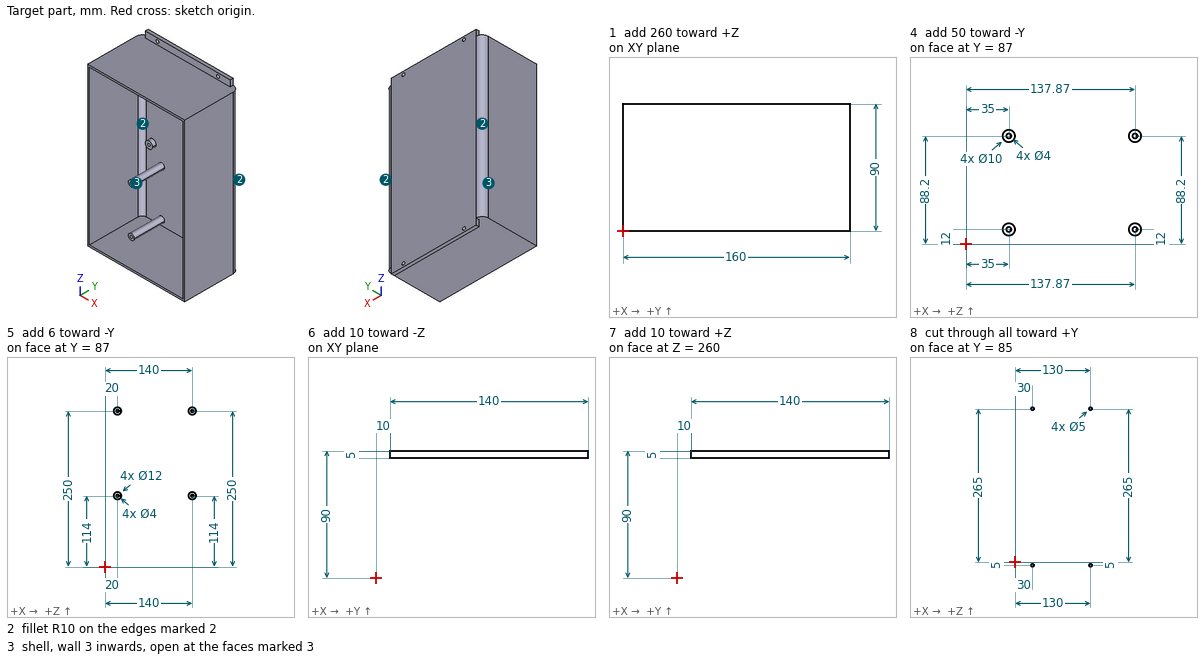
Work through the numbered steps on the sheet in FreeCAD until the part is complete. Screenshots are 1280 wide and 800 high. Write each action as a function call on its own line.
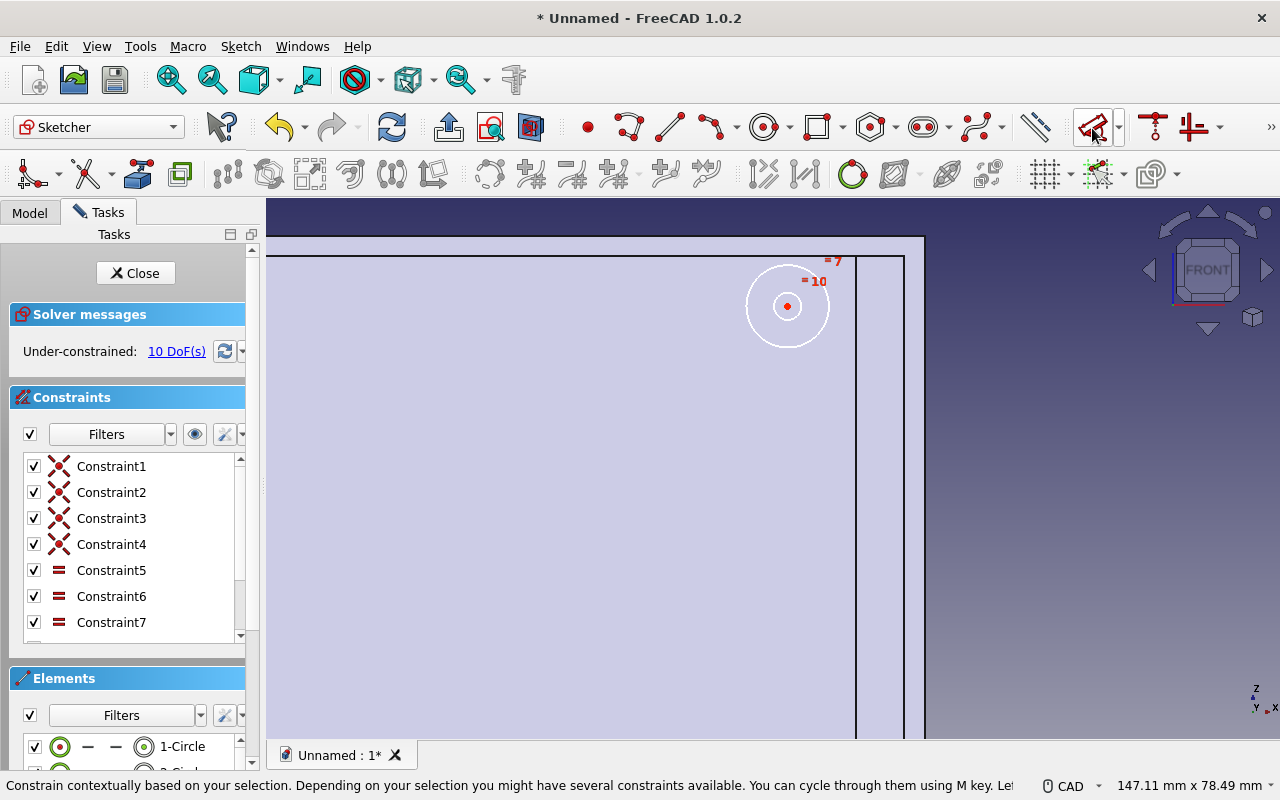
scroll(800, 297, down, 8)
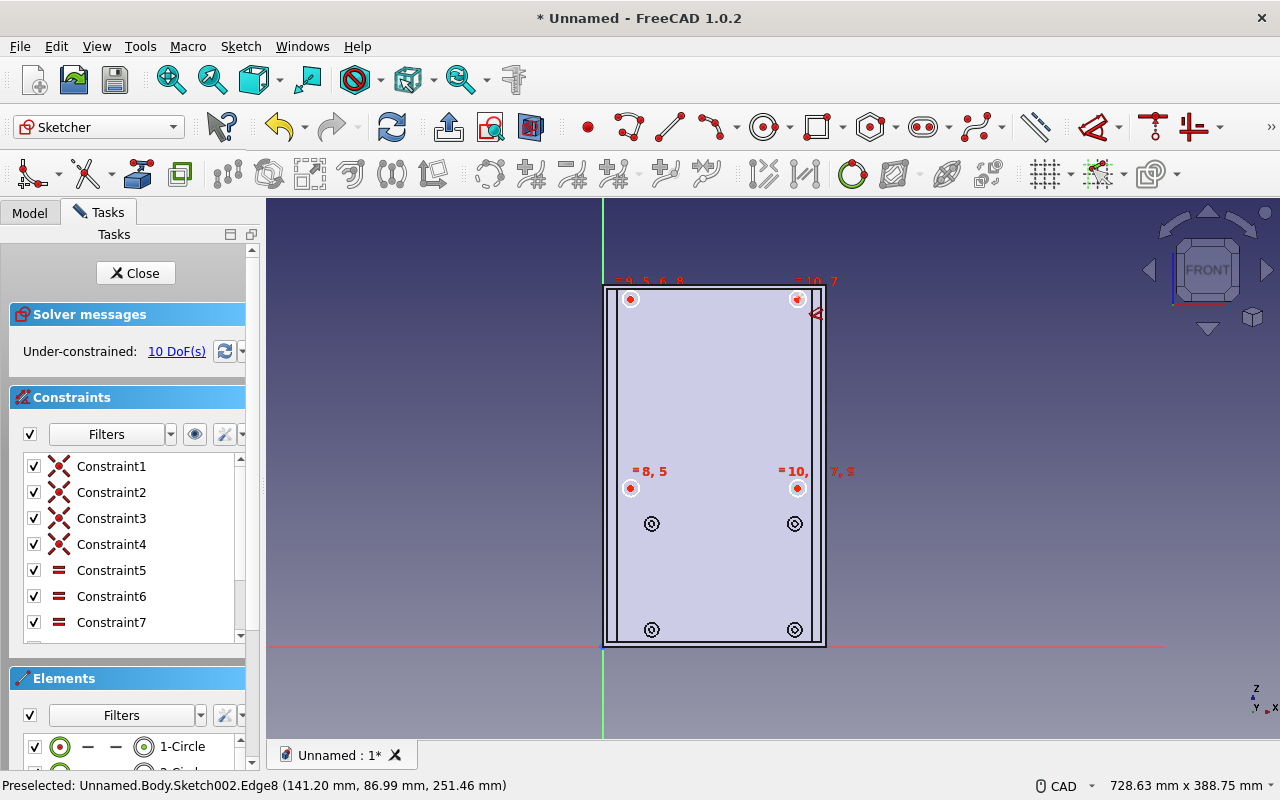
scroll(637, 482, up, 5)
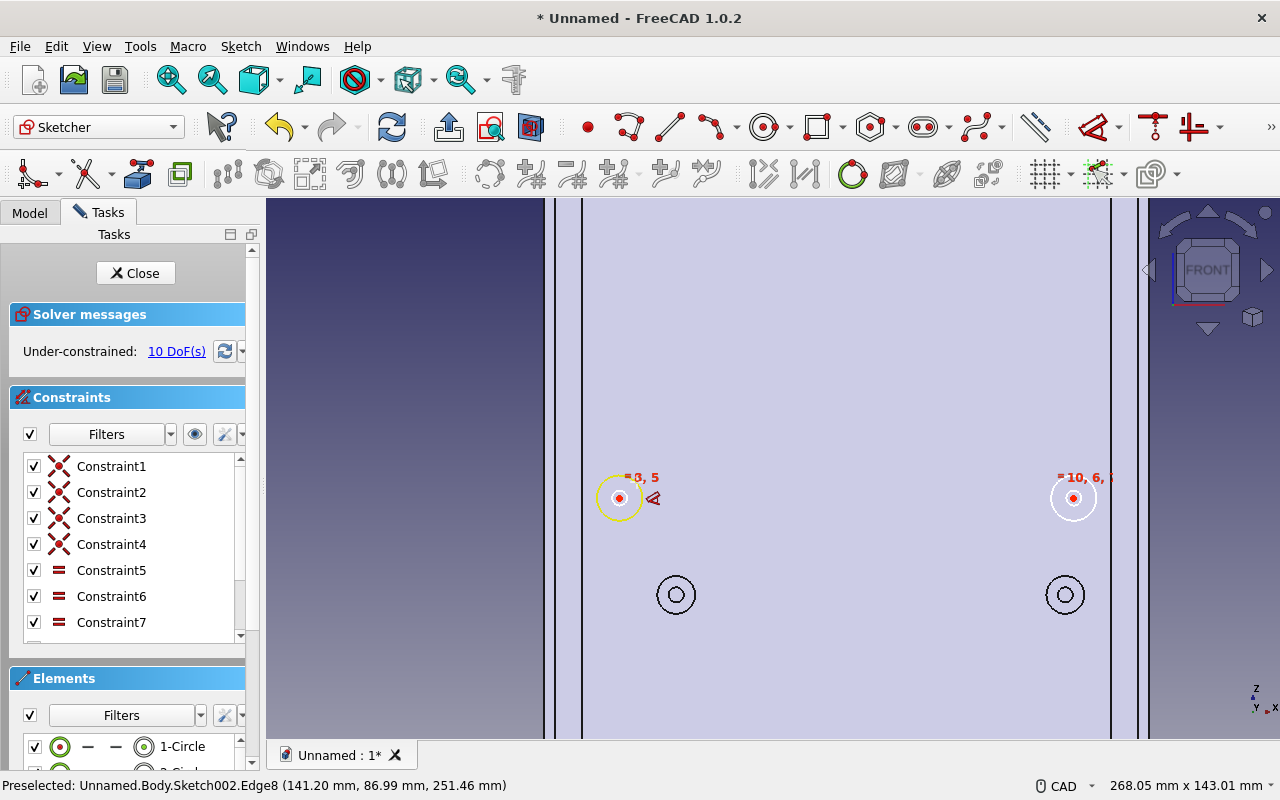
click(636, 482)
click(659, 460)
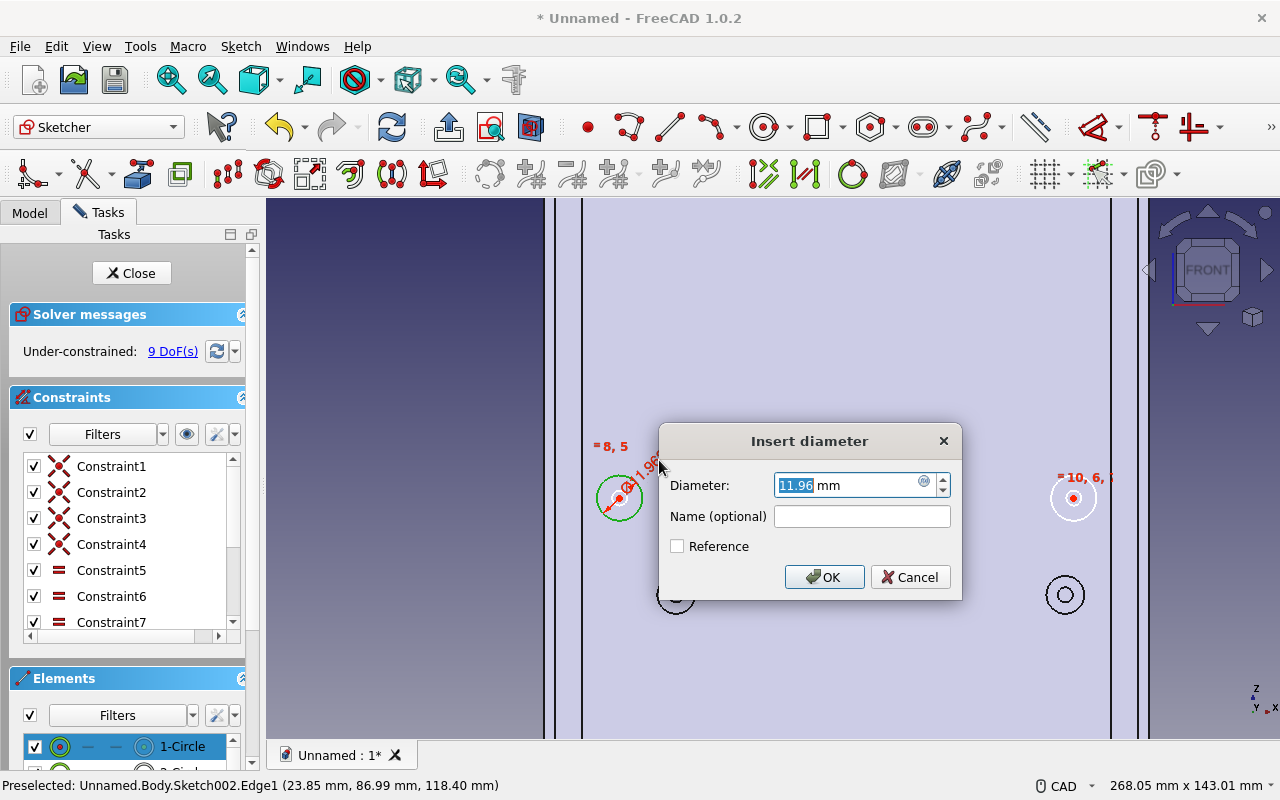
text(12)
key(Return)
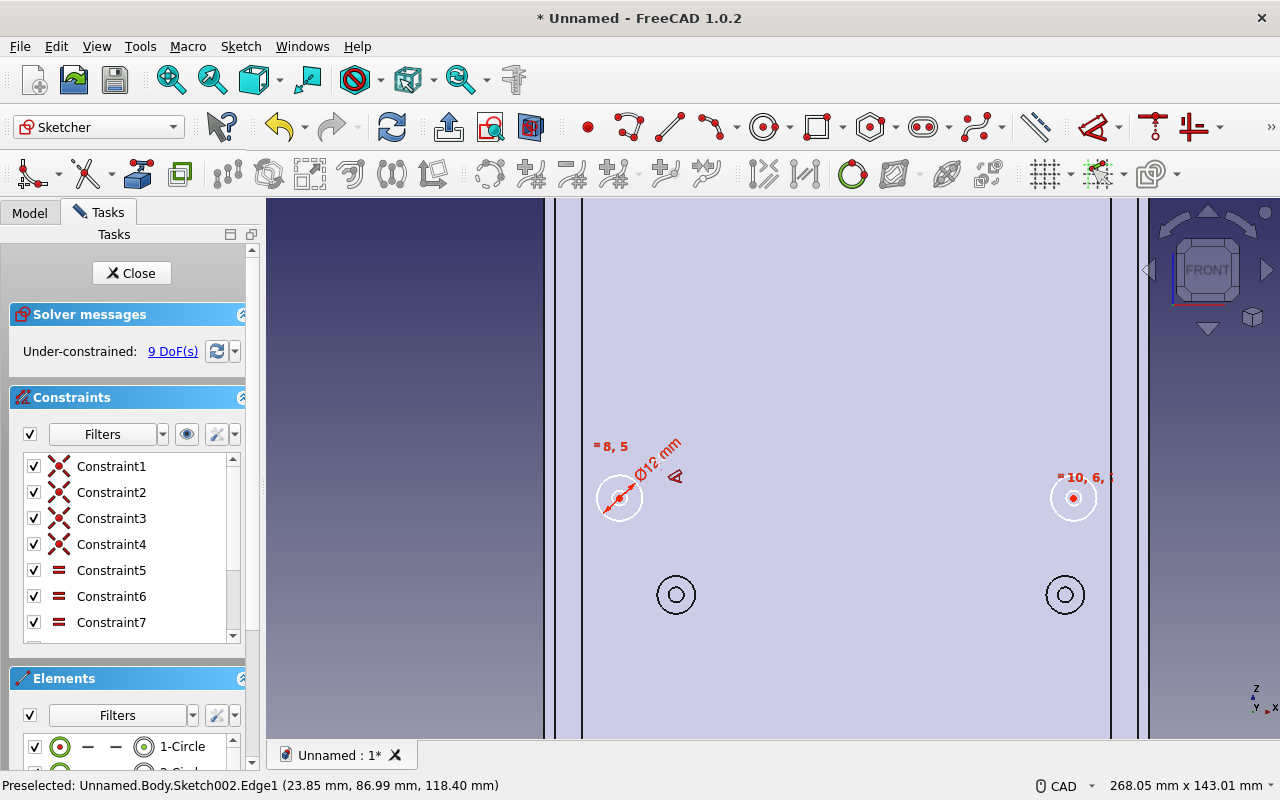
scroll(614, 493, up, 5)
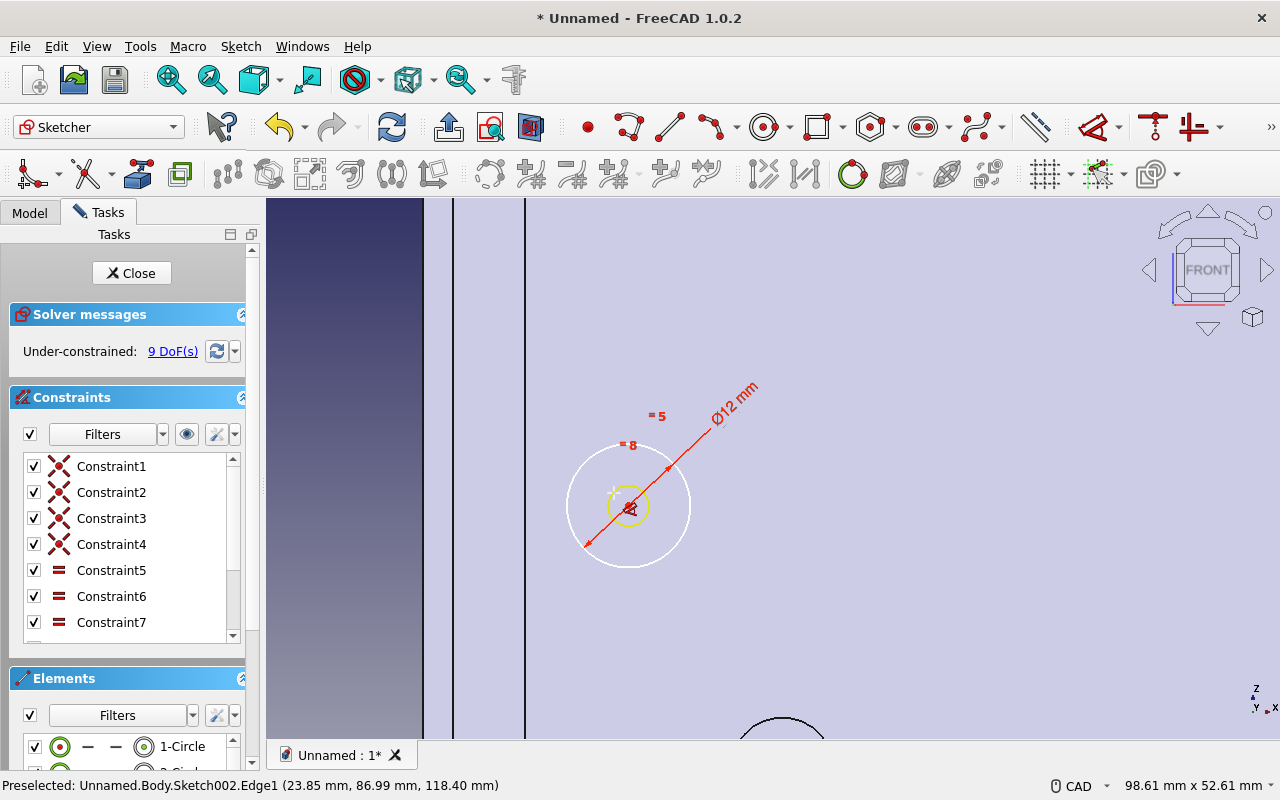
click(614, 492)
click(574, 454)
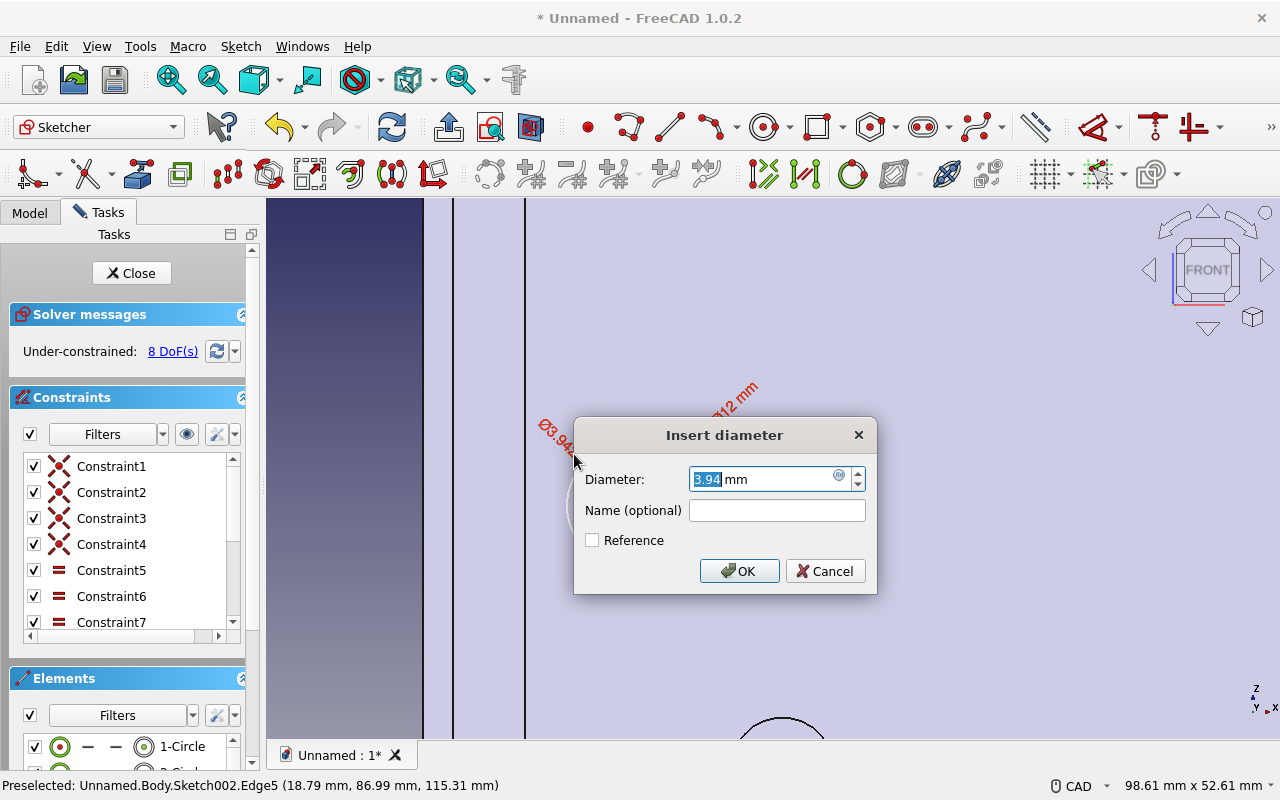
text(4)
key(Return)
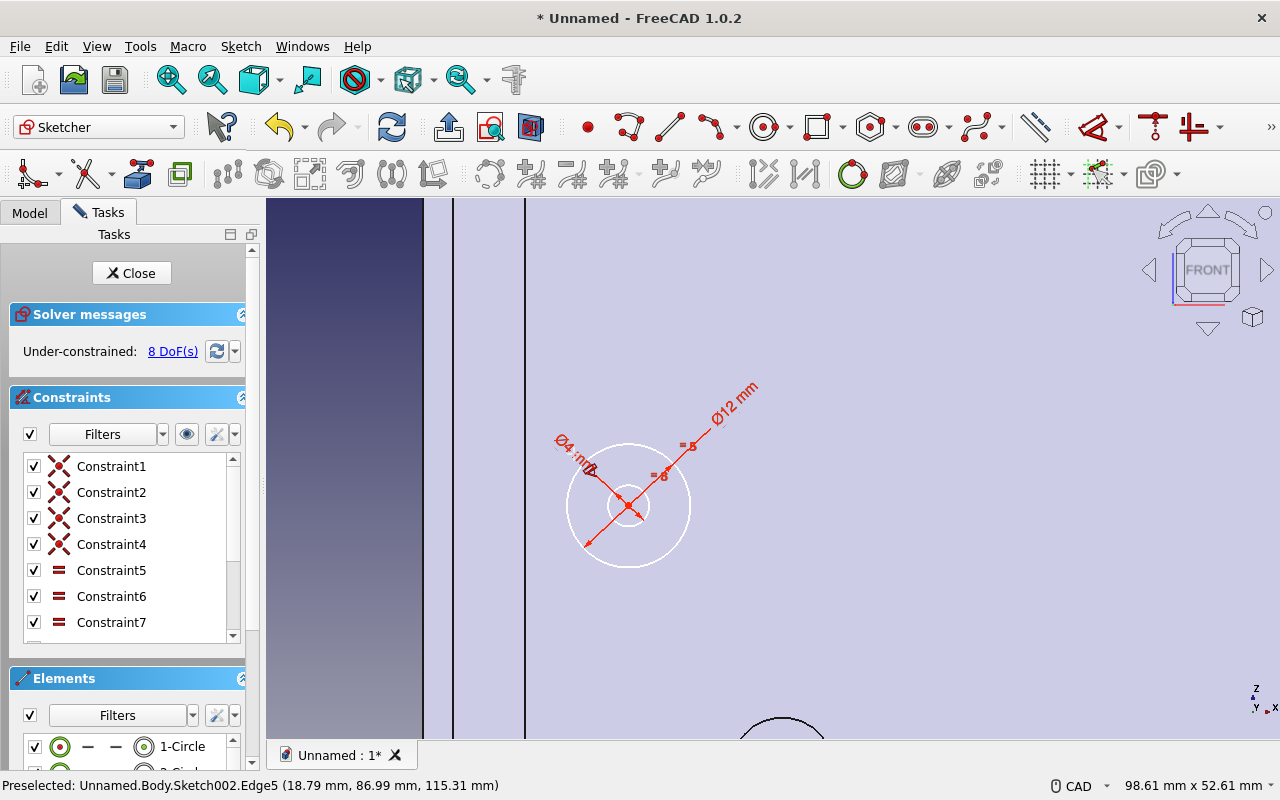
scroll(631, 486, down, 10)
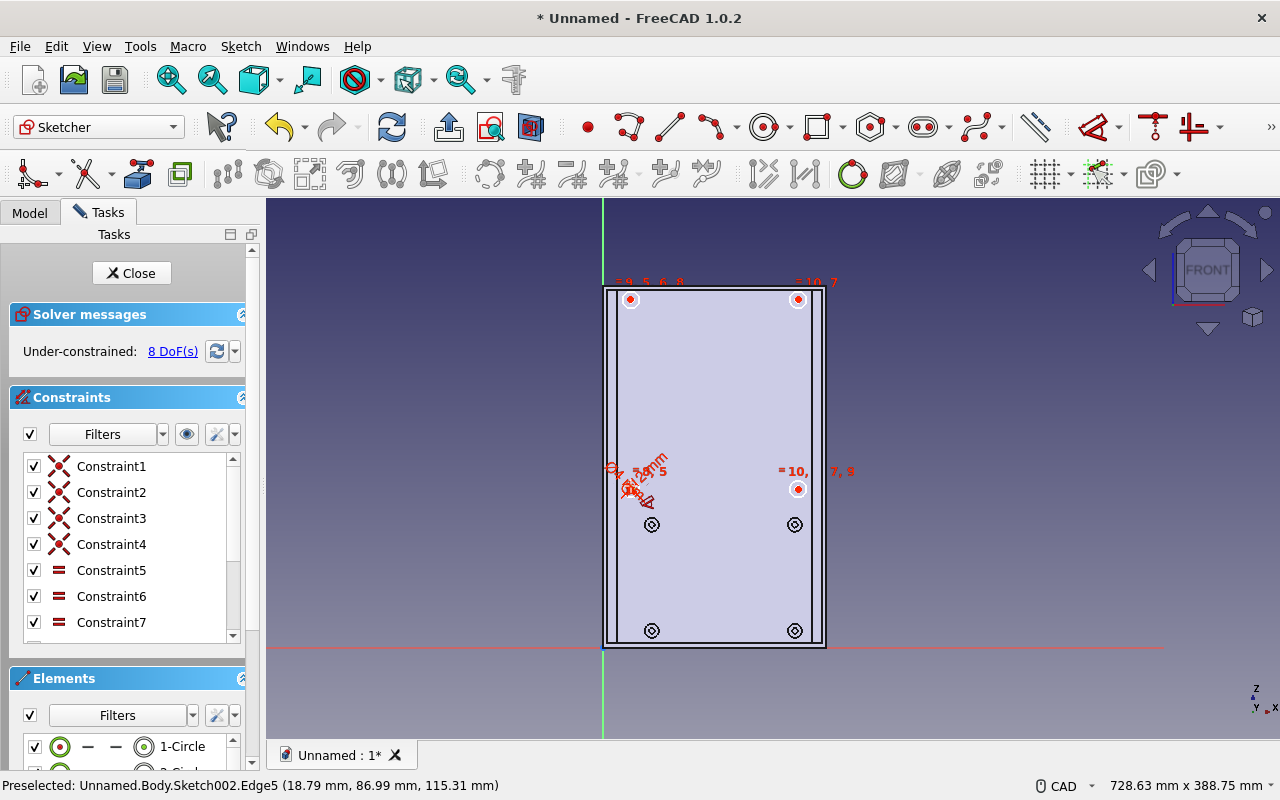
scroll(631, 489, up, 2)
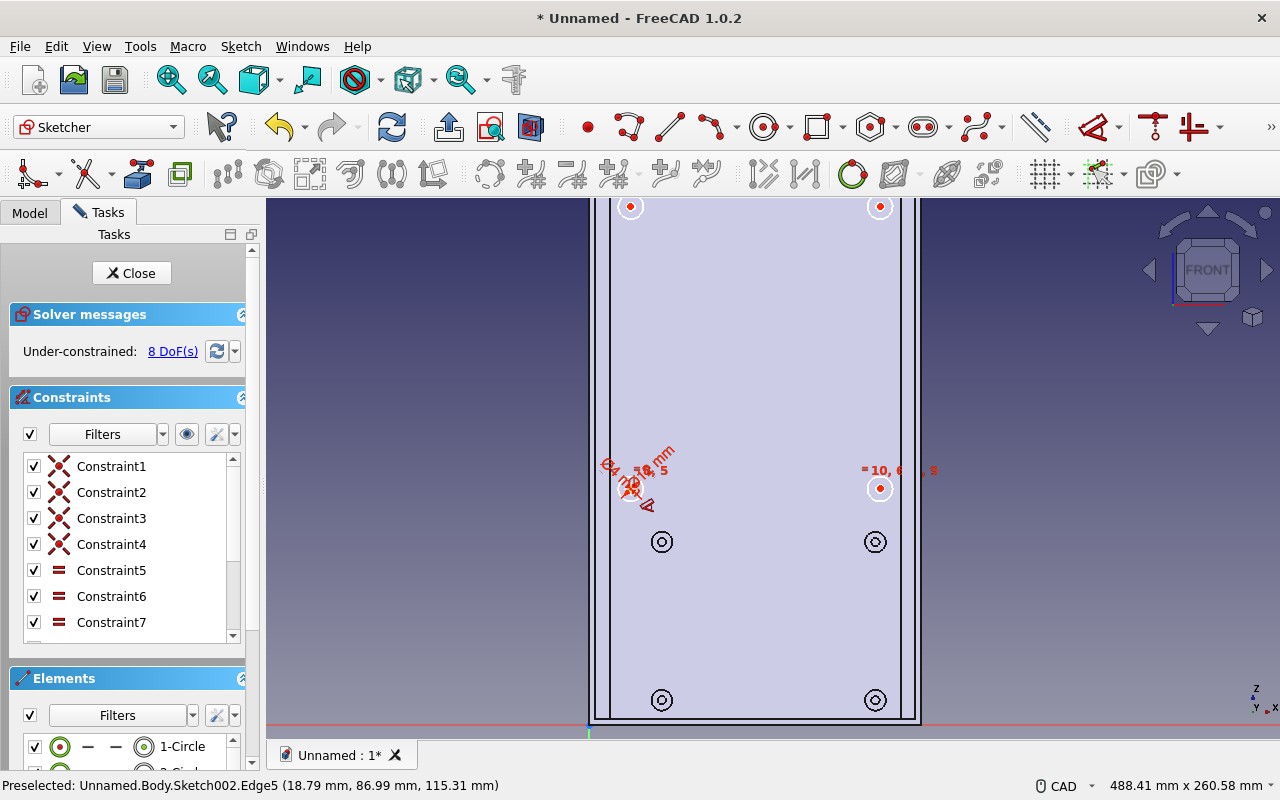
click(631, 489)
click(610, 431)